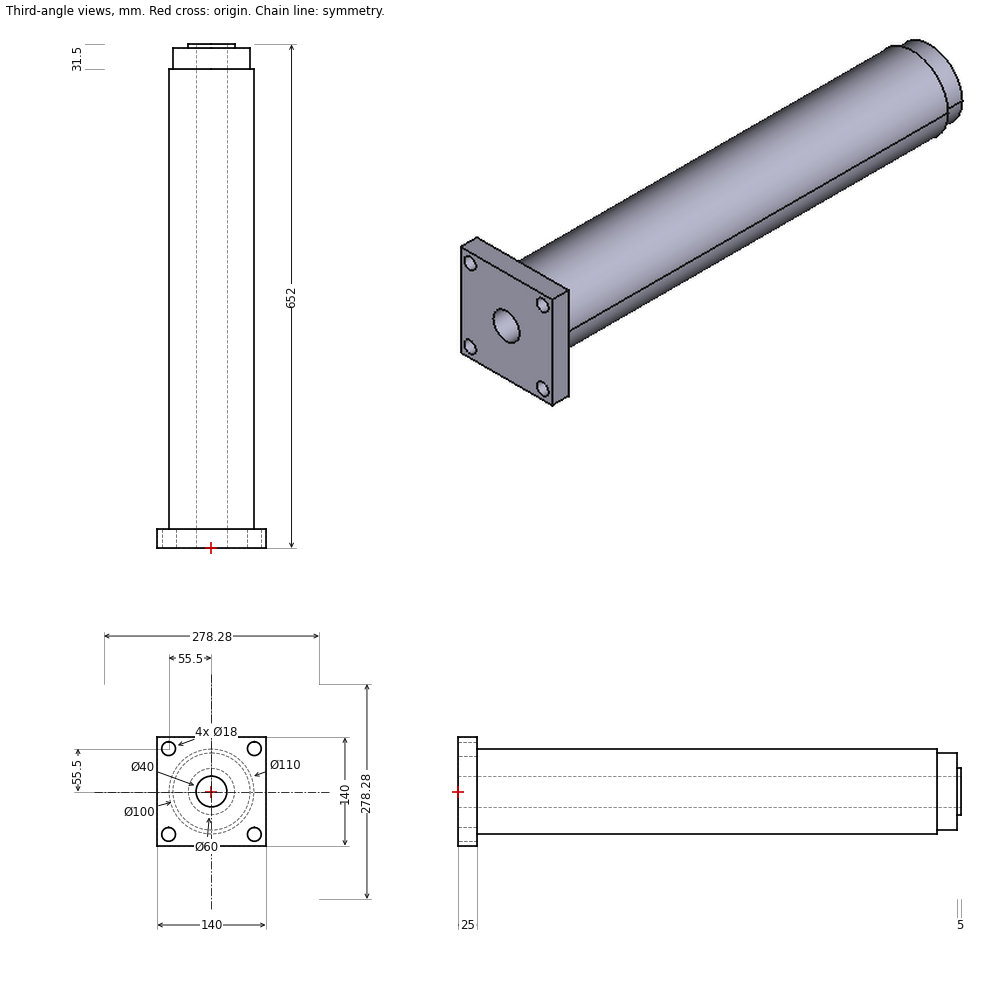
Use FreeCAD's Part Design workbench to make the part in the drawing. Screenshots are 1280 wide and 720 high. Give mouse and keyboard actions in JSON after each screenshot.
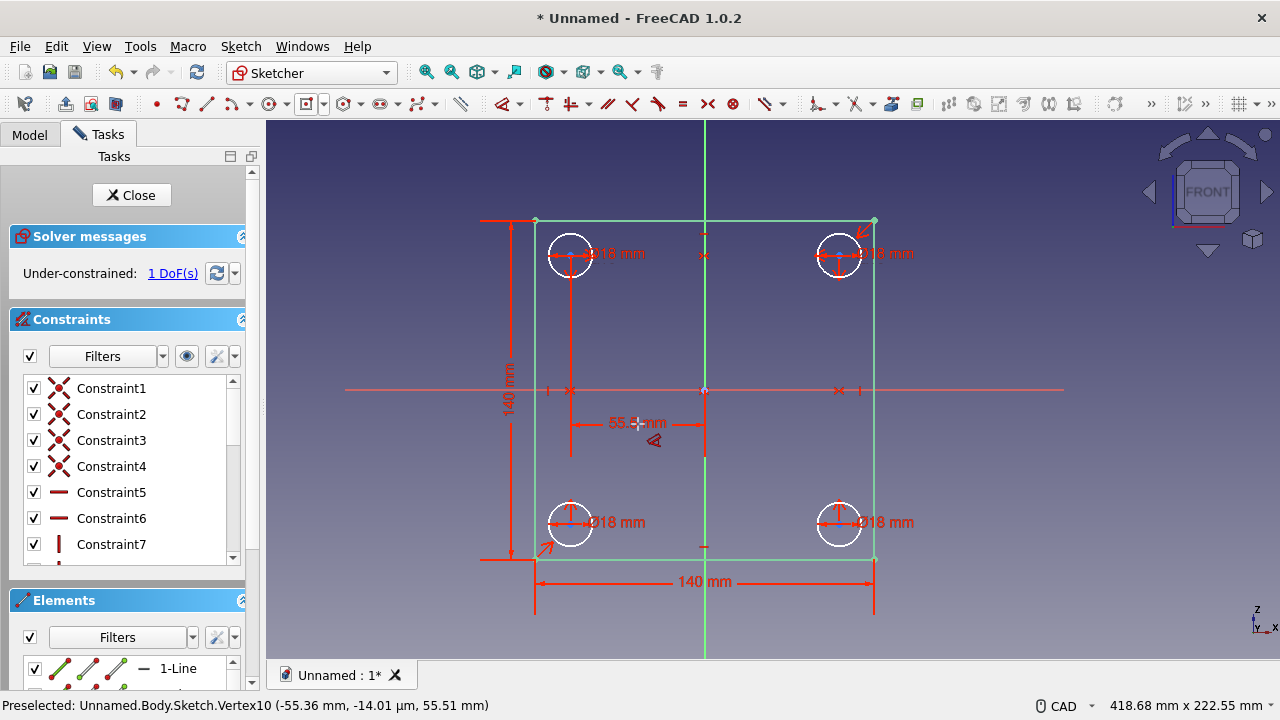
{"action": "left_click", "coordinate": [571, 256]}
{"action": "left_click", "coordinate": [739, 323]}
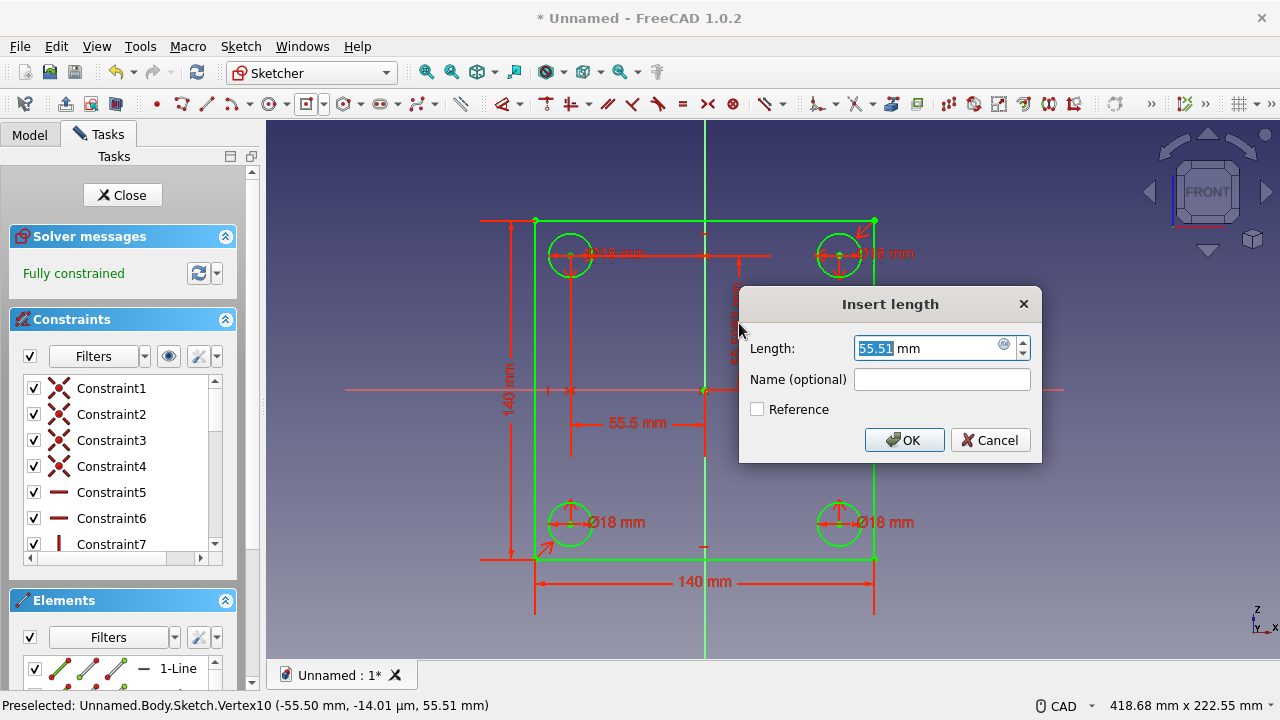
{"action": "type", "text": "55.5"}
{"action": "key", "text": "Return"}
{"action": "key", "text": "Escape"}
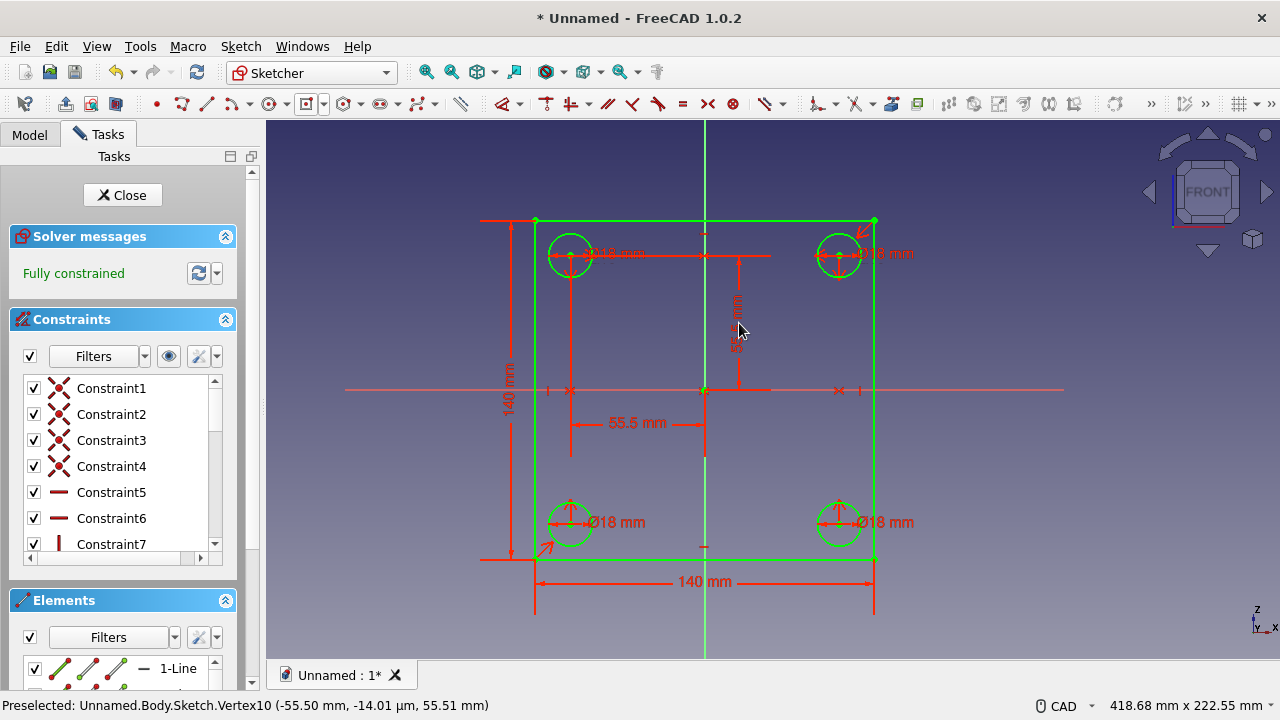
{"action": "left_click", "coordinate": [123, 195]}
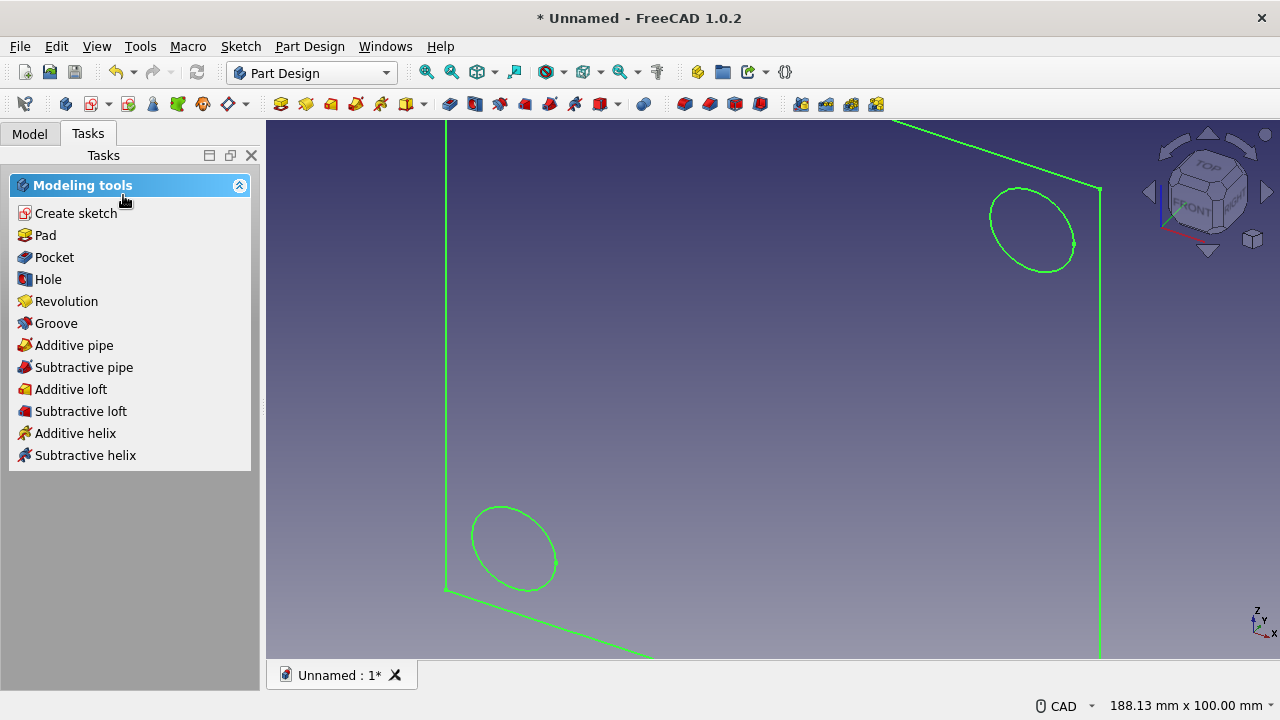
{"action": "left_click", "coordinate": [281, 104]}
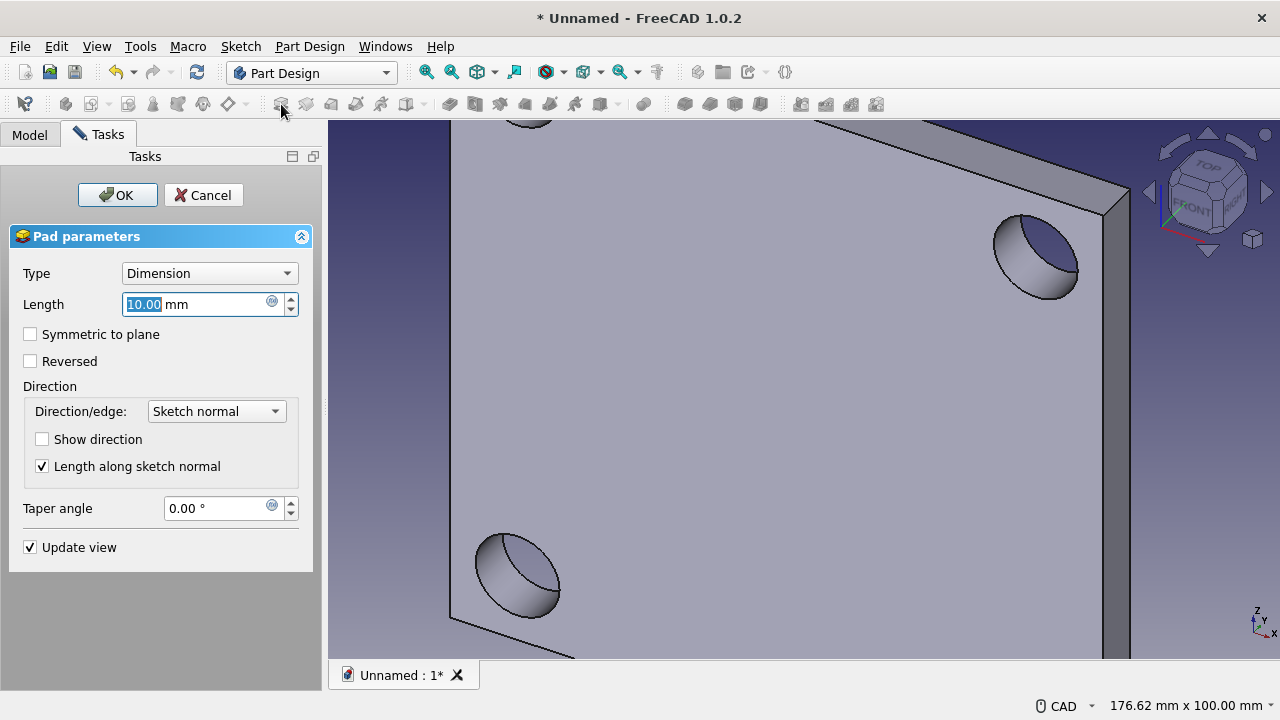
{"action": "type", "text": "25"}
{"action": "key", "text": "Tab"}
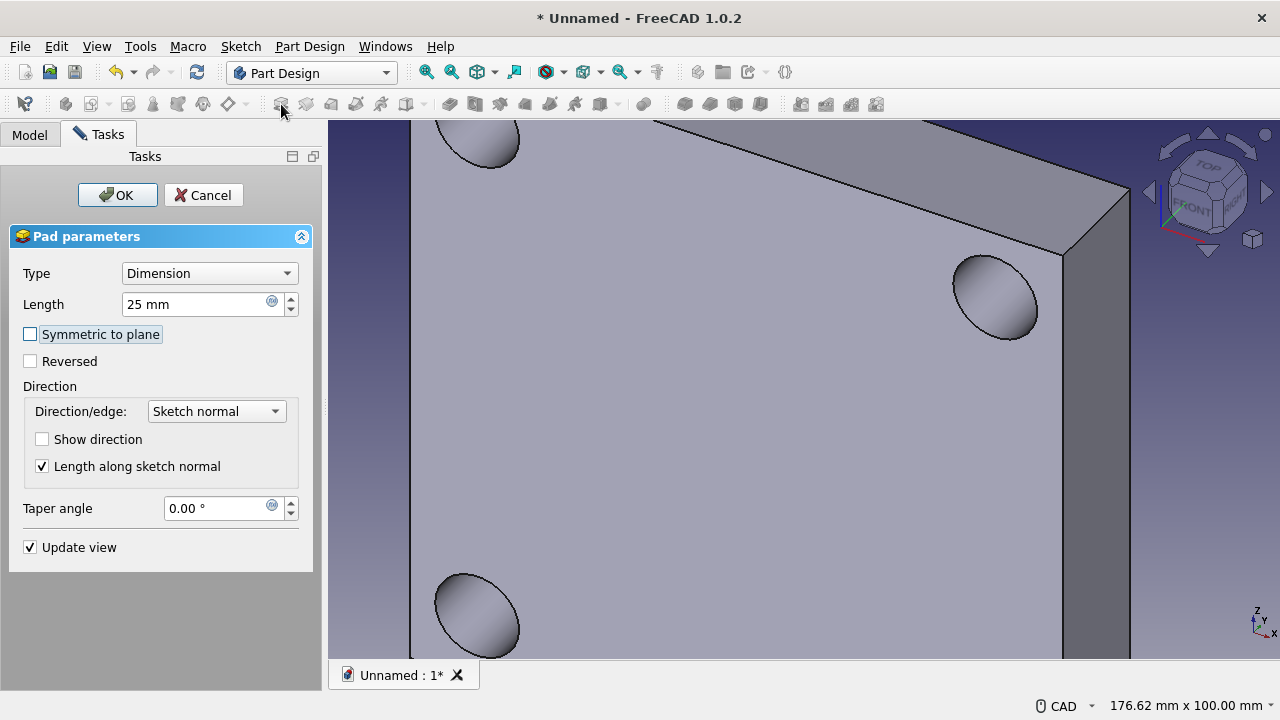
{"action": "left_click", "coordinate": [31, 361]}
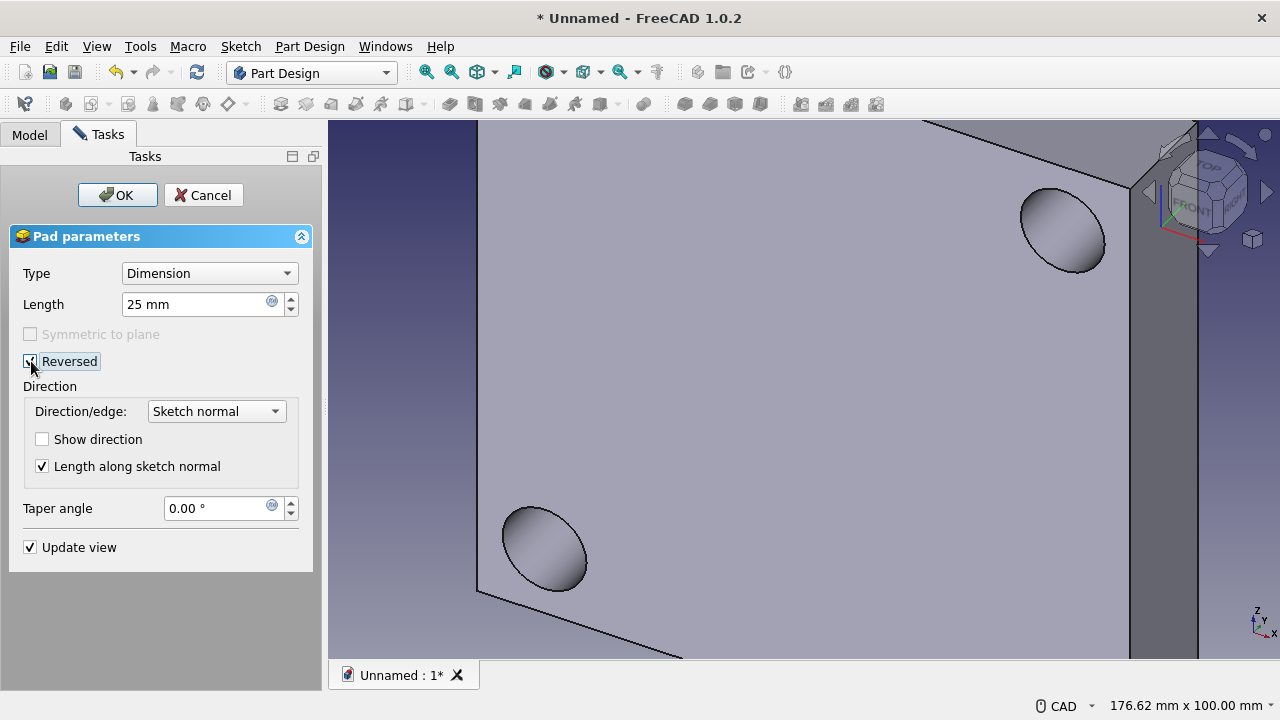
{"action": "left_click", "coordinate": [118, 195]}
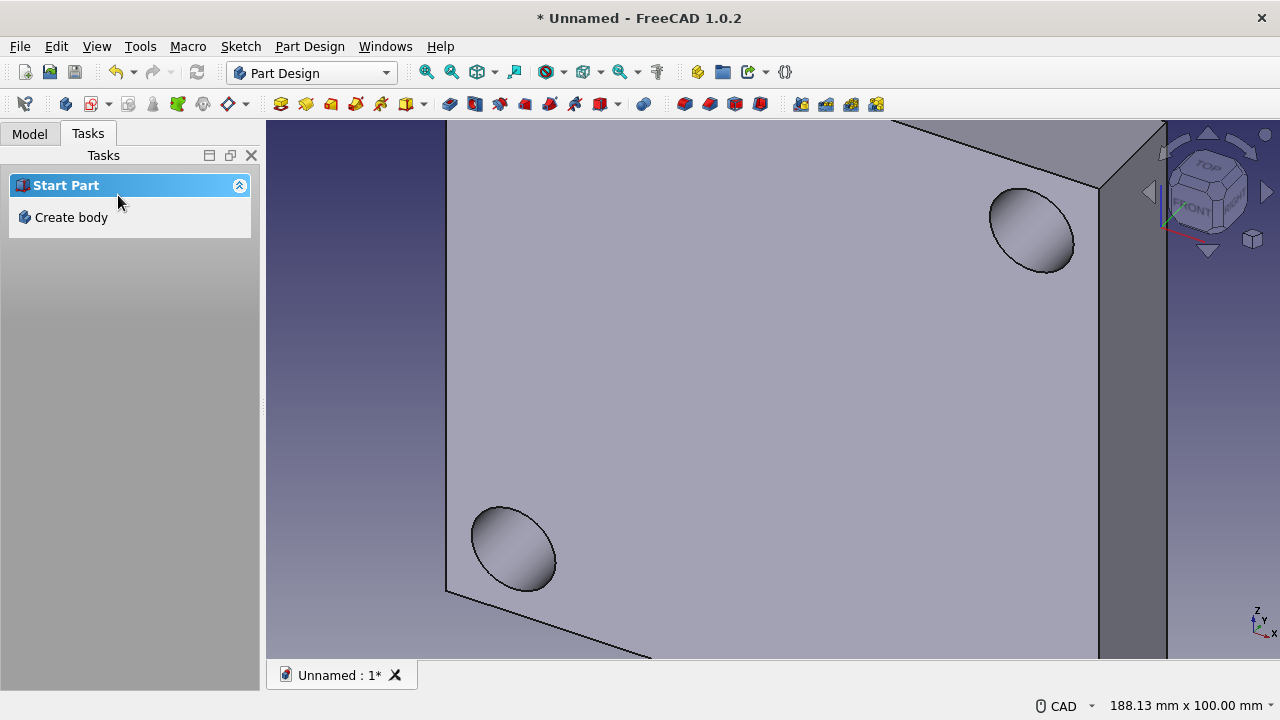
{"action": "left_click", "coordinate": [427, 72]}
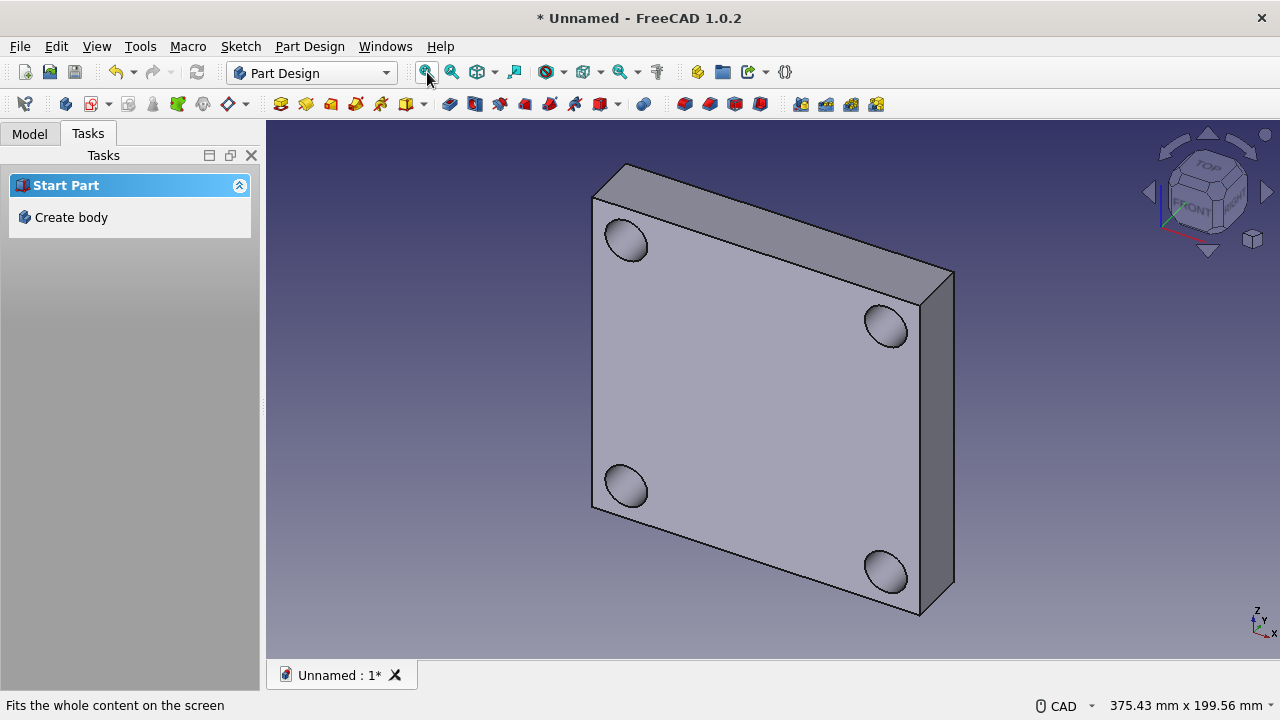
{"action": "left_click", "coordinate": [90, 104]}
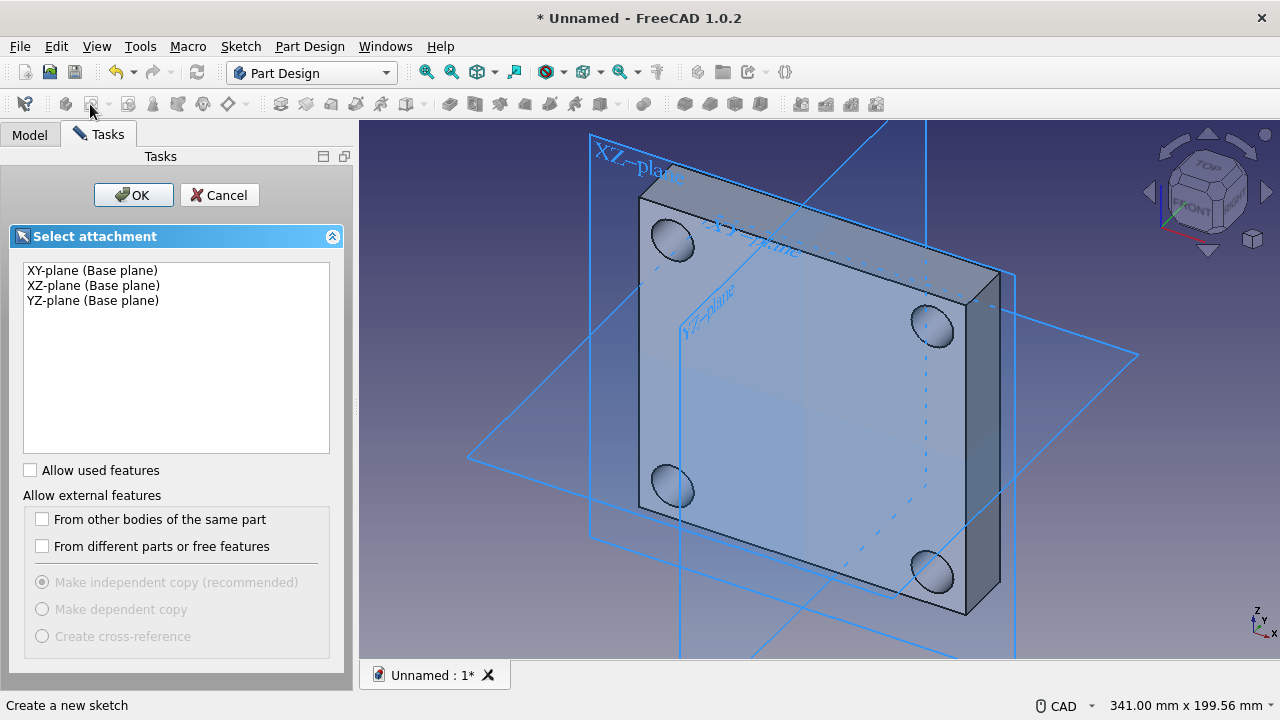
{"action": "left_click", "coordinate": [84, 286]}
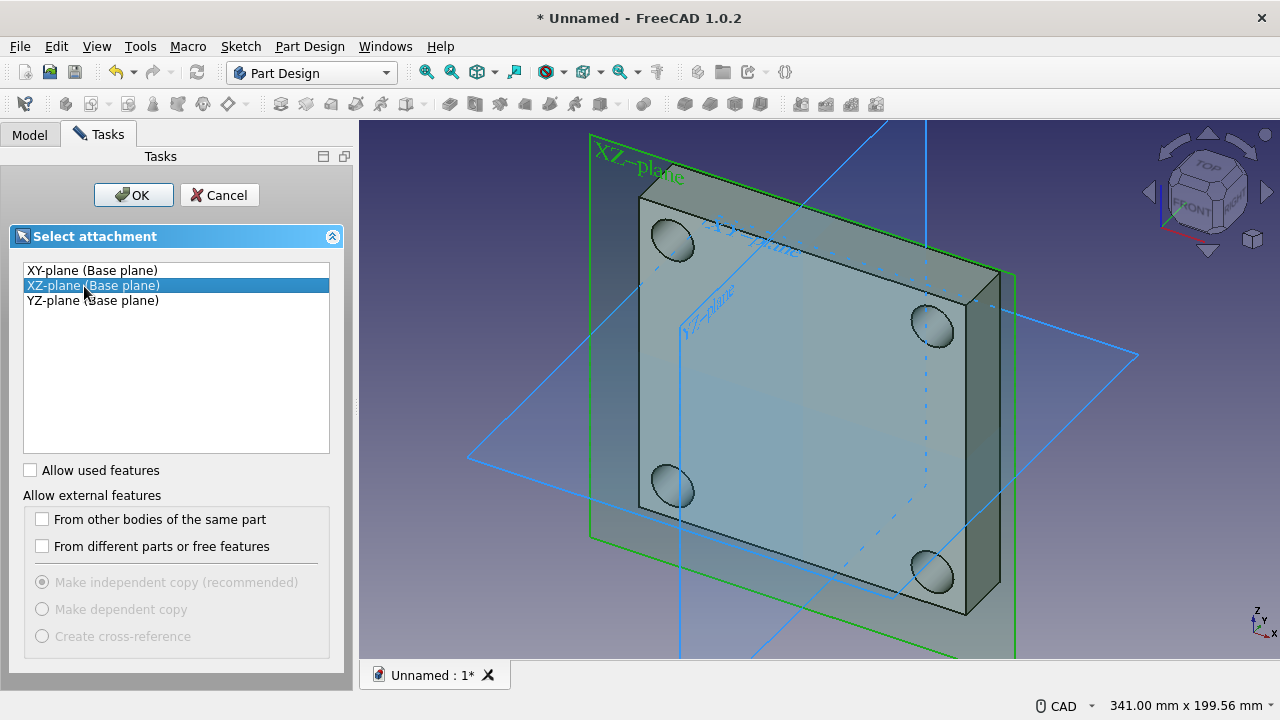
{"action": "left_click", "coordinate": [134, 195]}